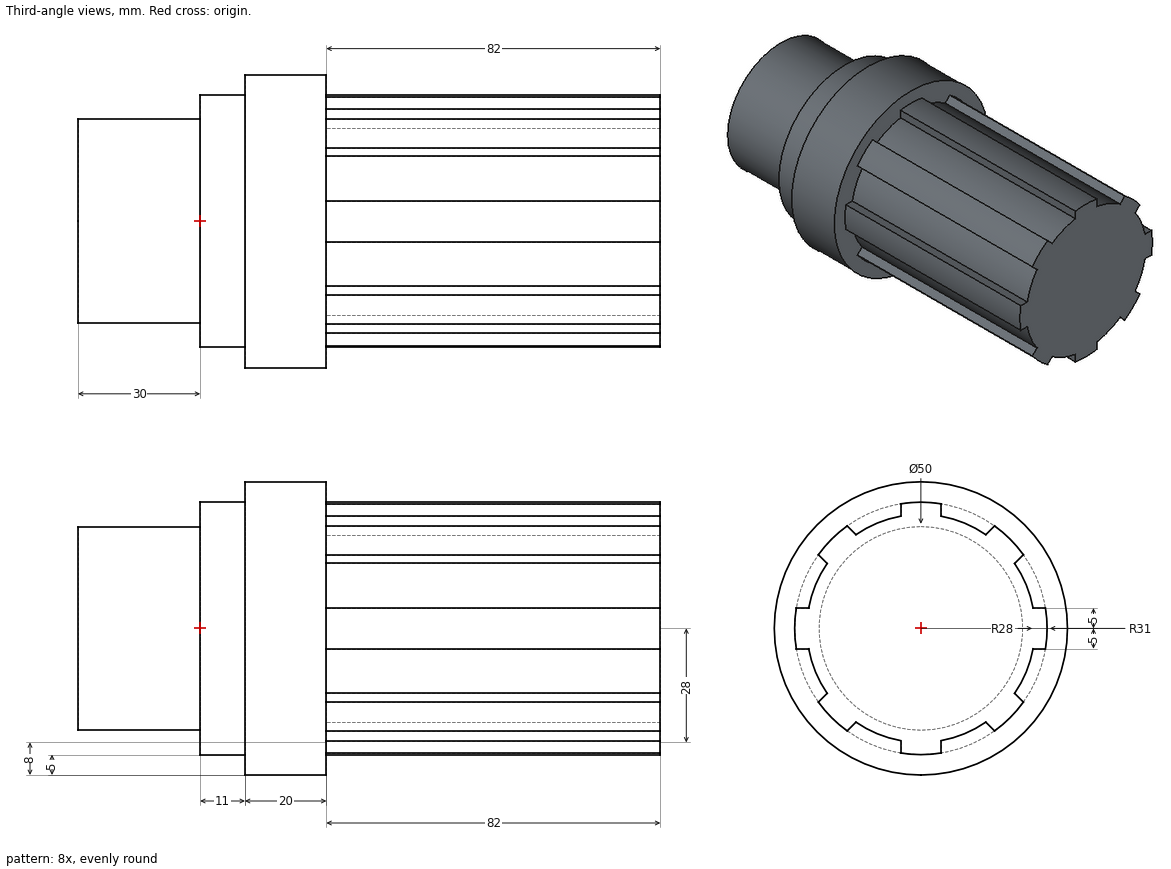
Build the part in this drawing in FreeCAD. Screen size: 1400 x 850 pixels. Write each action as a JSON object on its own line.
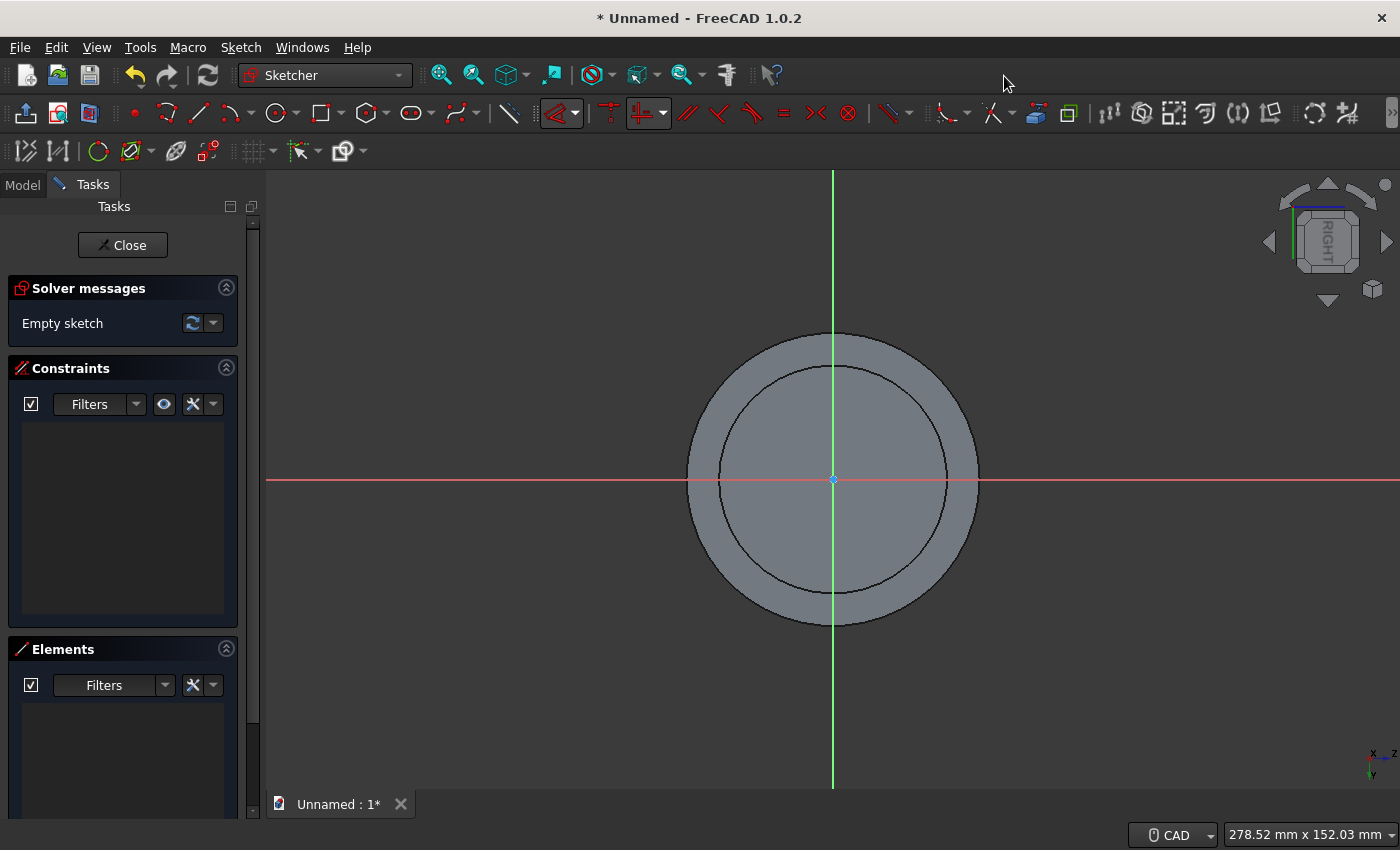
{"action": "scroll", "coordinate": [837, 606], "scroll_direction": "up", "scroll_amount": 14}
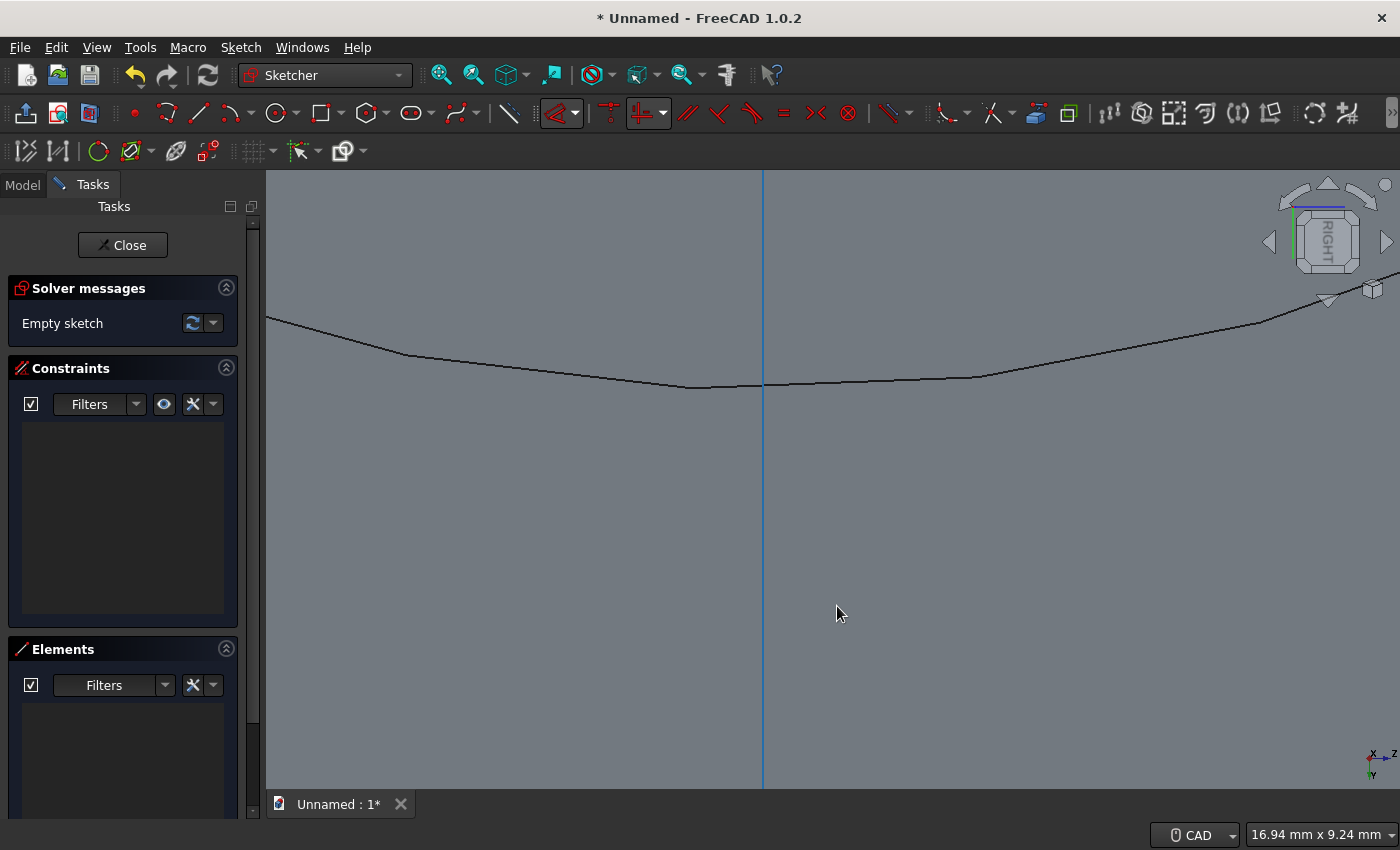
{"action": "left_click", "coordinate": [200, 114]}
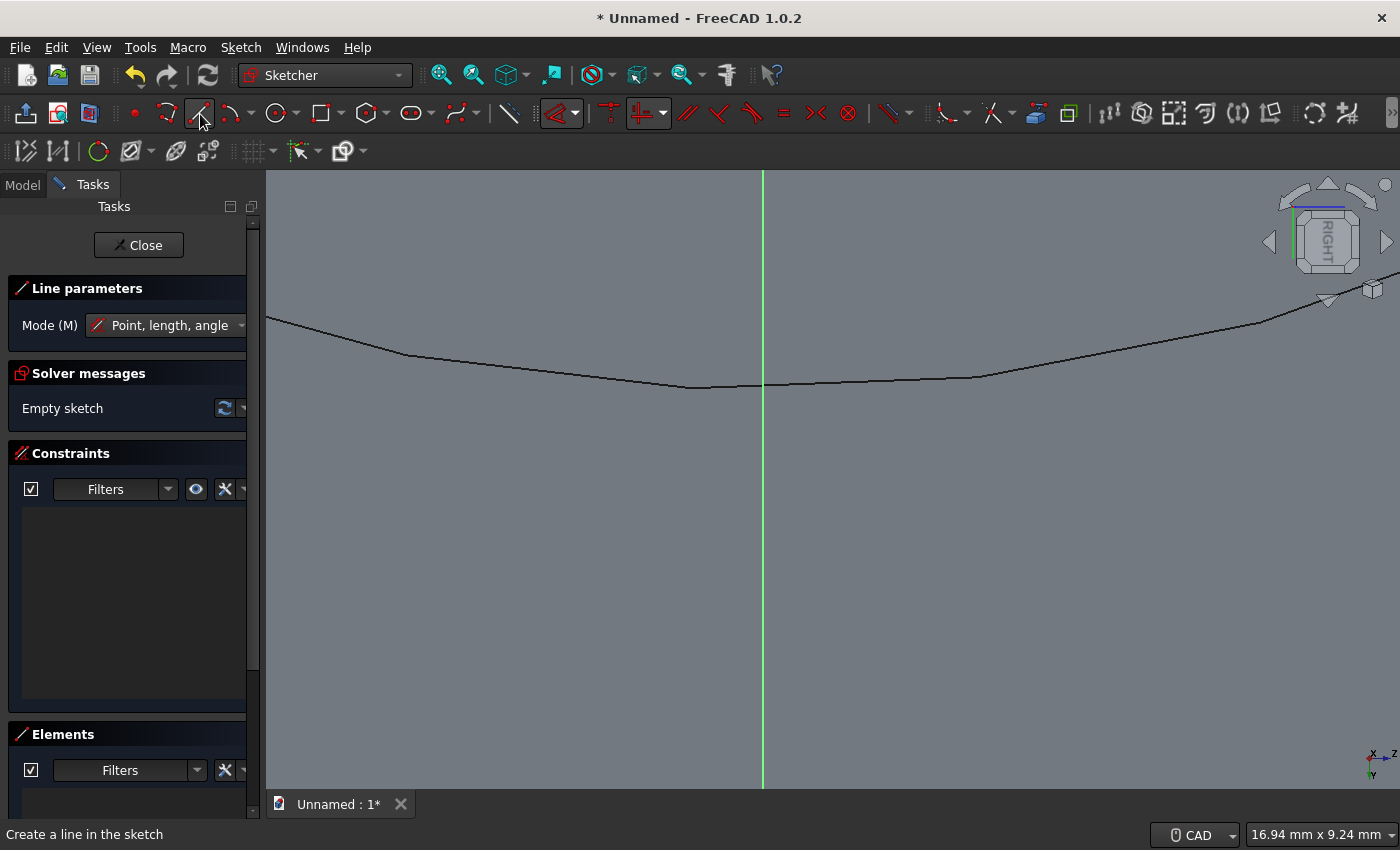
{"action": "left_click", "coordinate": [1098, 563]}
{"action": "left_click", "coordinate": [1098, 359]}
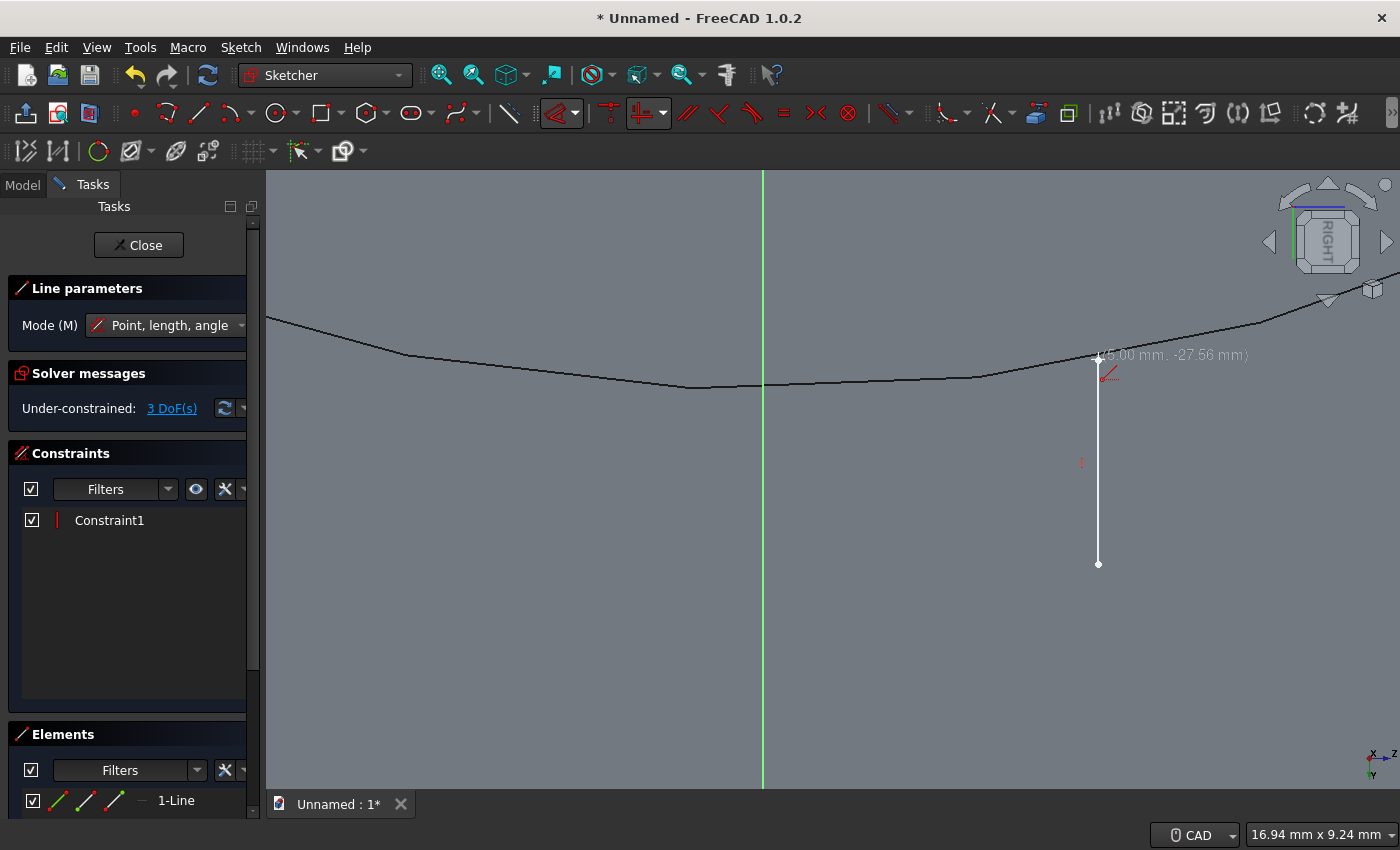
{"action": "left_click", "coordinate": [429, 359]}
{"action": "left_click", "coordinate": [429, 563]}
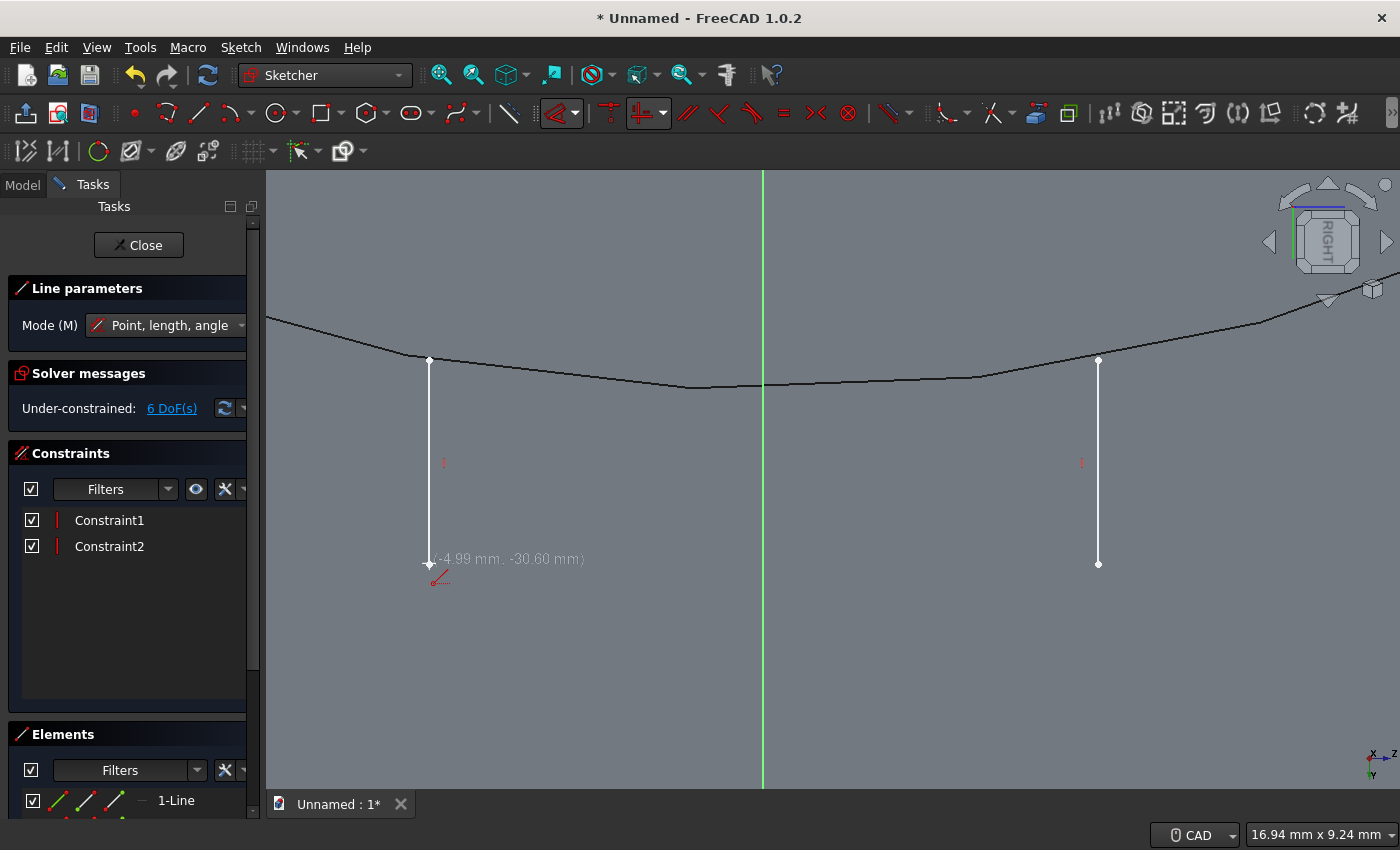
{"action": "key", "text": "g 3 a"}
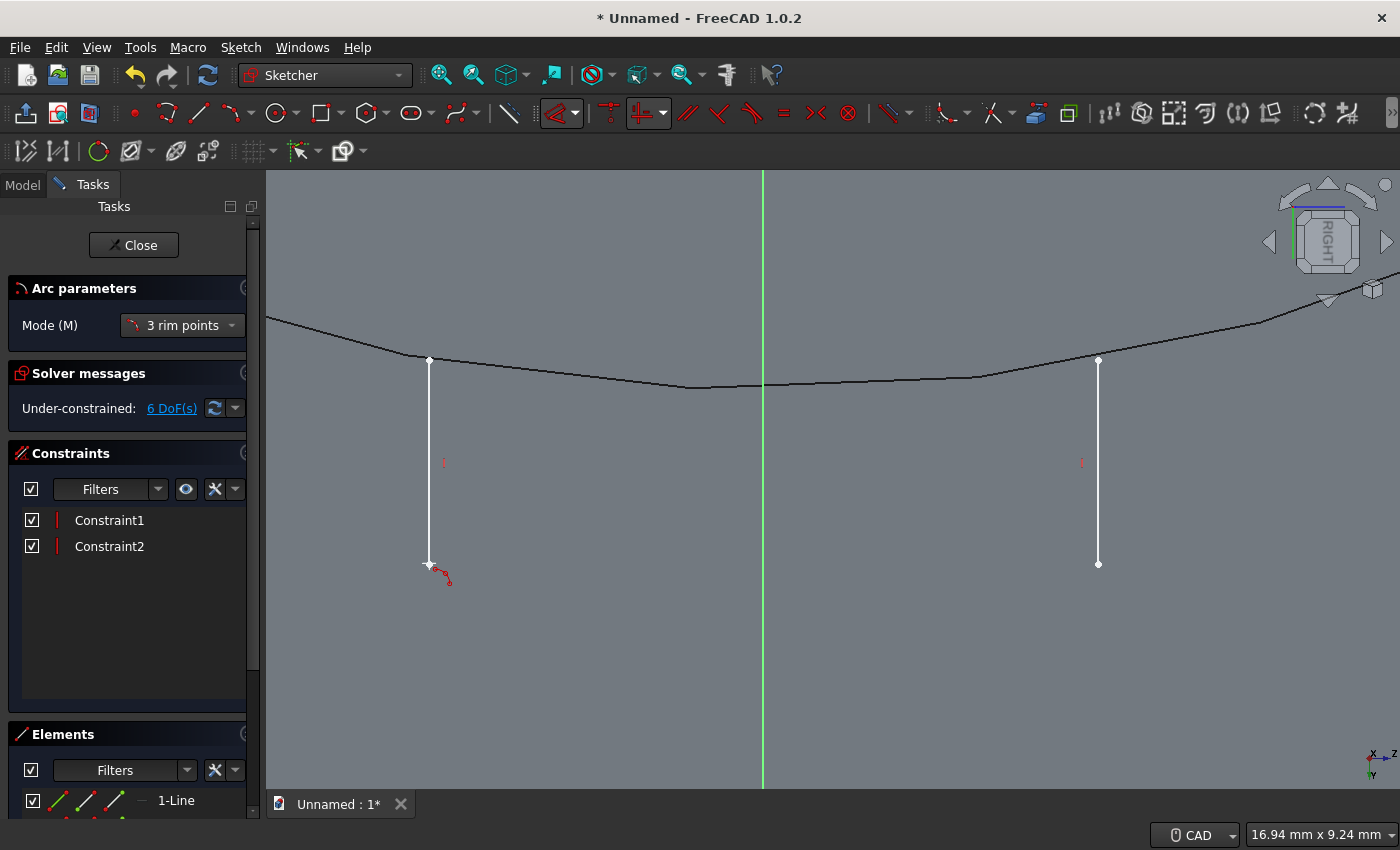
{"action": "left_click", "coordinate": [1098, 360]}
{"action": "left_click", "coordinate": [429, 360]}
{"action": "left_click", "coordinate": [696, 388]}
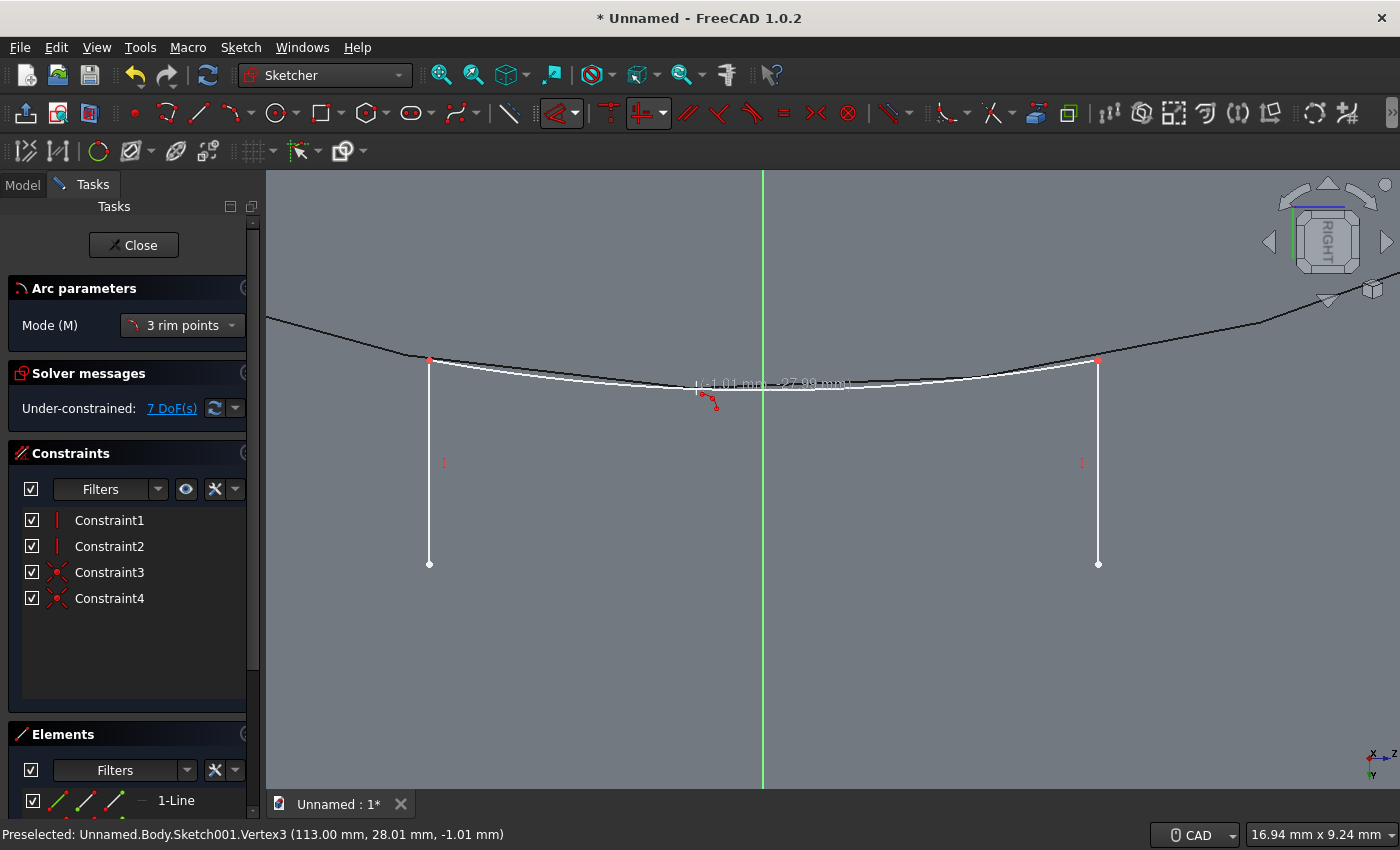
{"action": "left_click", "coordinate": [429, 564]}
{"action": "left_click", "coordinate": [1098, 564]}
{"action": "left_click", "coordinate": [696, 589]}
{"action": "key", "text": "Escape"}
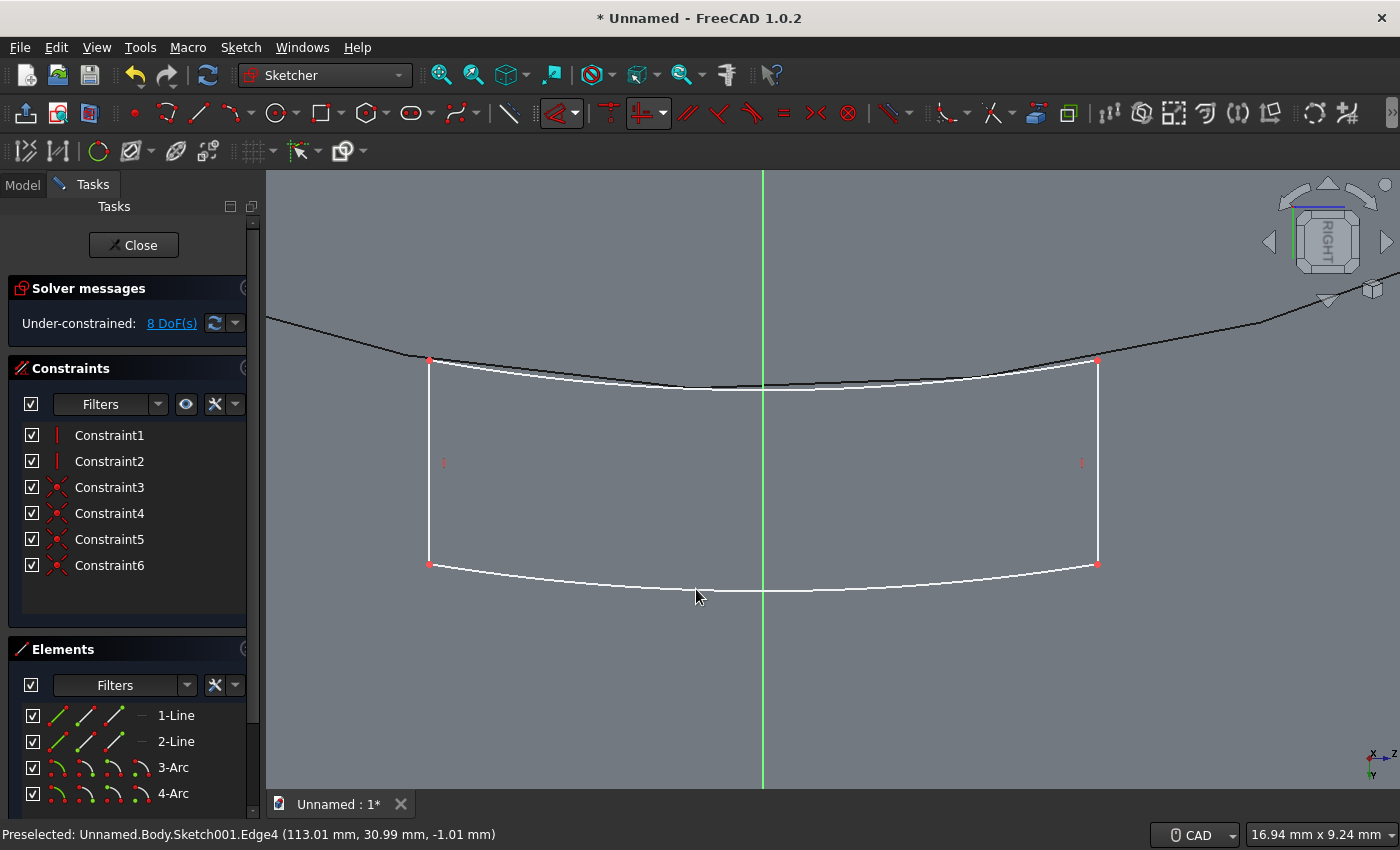
{"action": "left_click", "coordinate": [629, 385]}